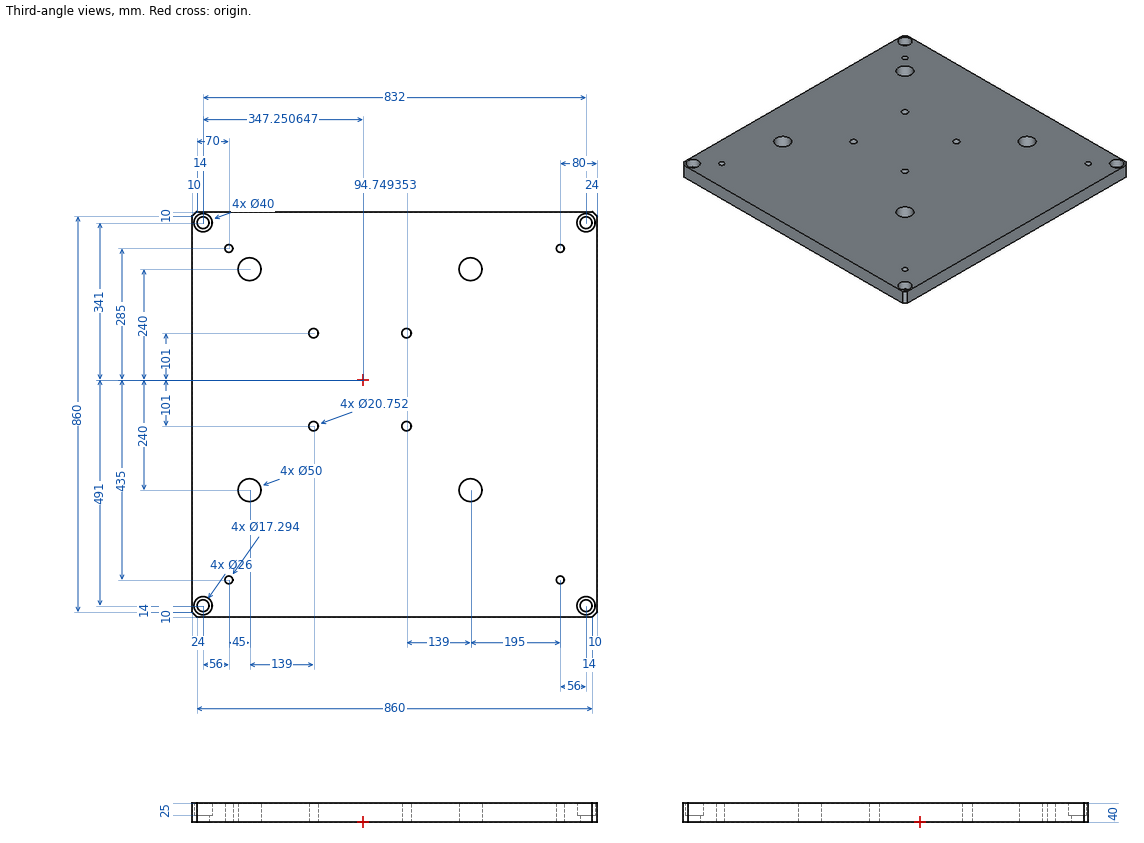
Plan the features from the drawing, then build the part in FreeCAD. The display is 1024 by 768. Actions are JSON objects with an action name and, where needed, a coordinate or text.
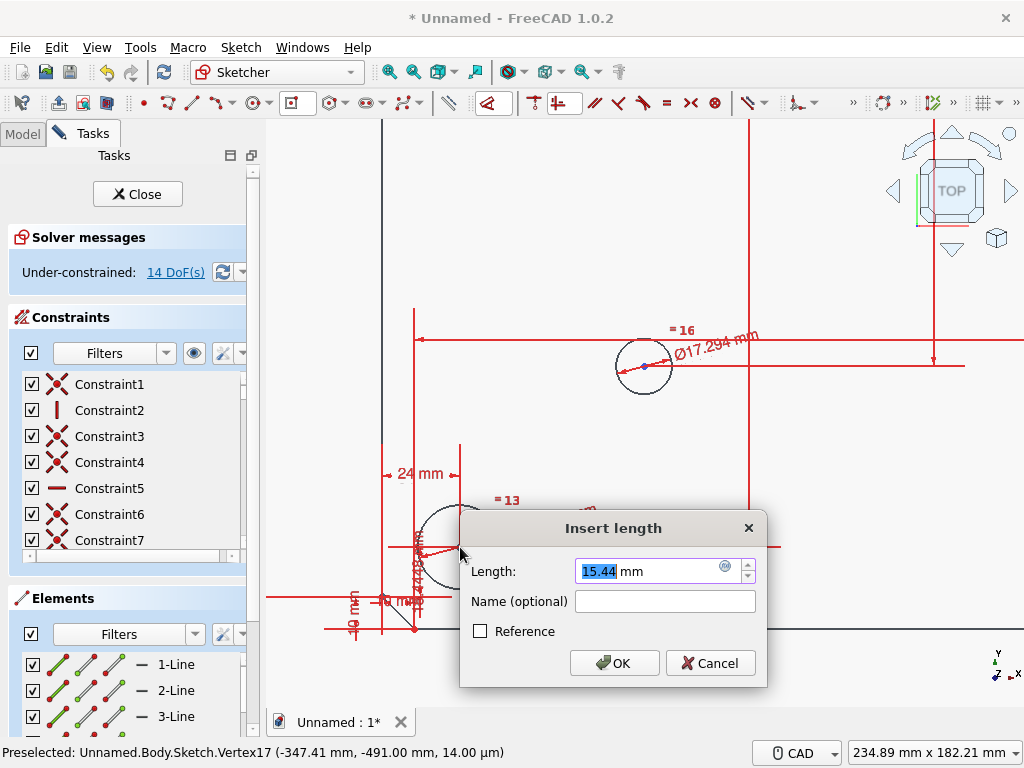
{"action": "type", "text": "14"}
{"action": "key", "text": "Return"}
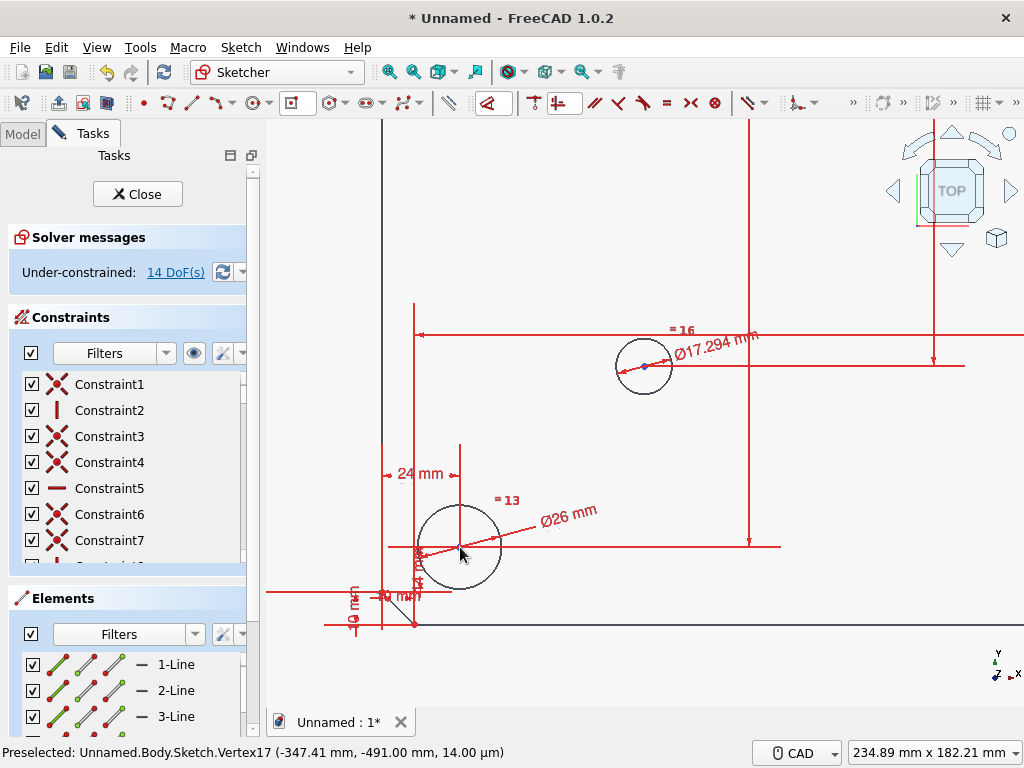
{"action": "scroll", "coordinate": [385, 602], "scroll_direction": "down", "scroll_amount": 10}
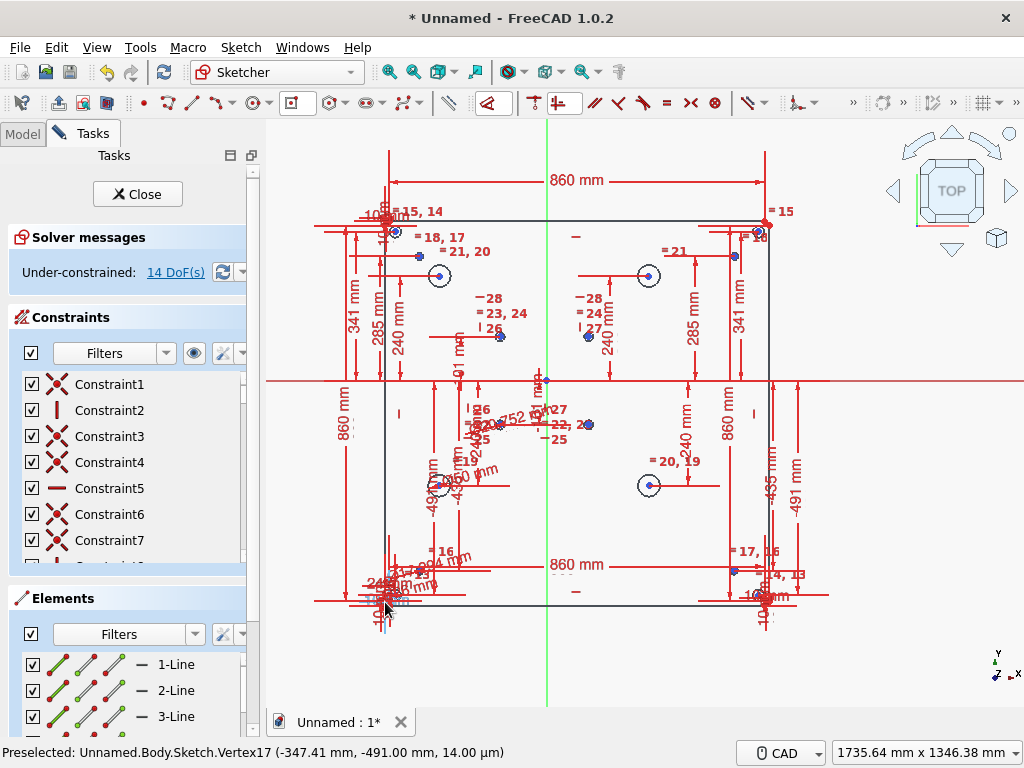
{"action": "scroll", "coordinate": [395, 595], "scroll_direction": "up", "scroll_amount": 3}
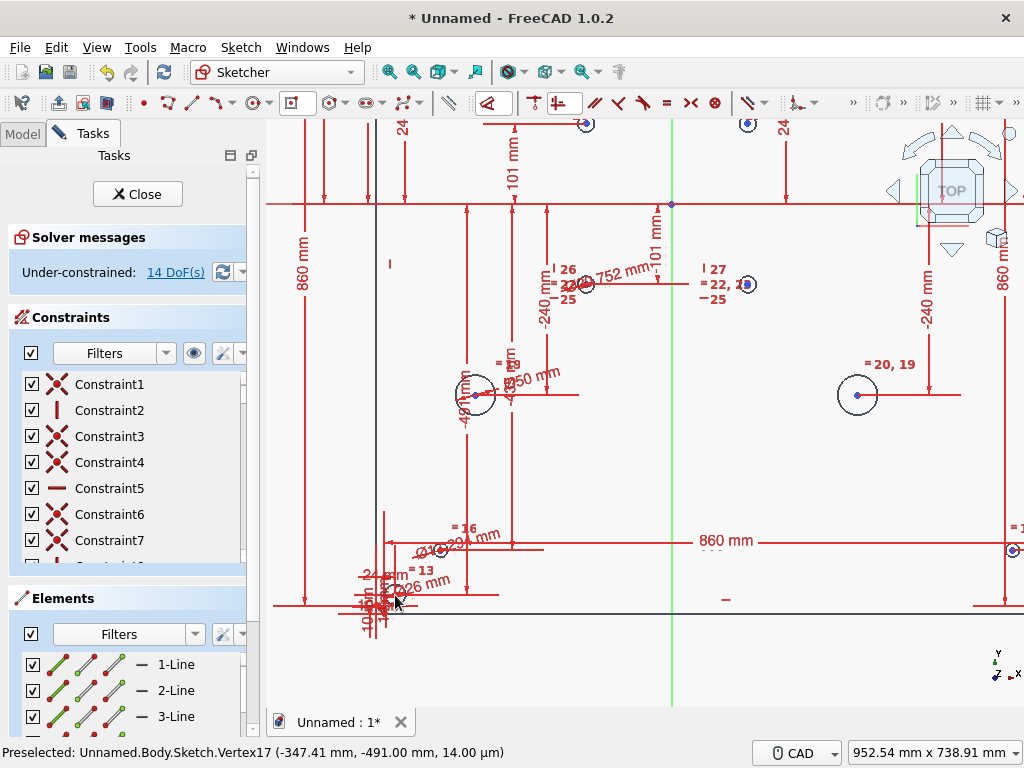
{"action": "left_click", "coordinate": [395, 595]}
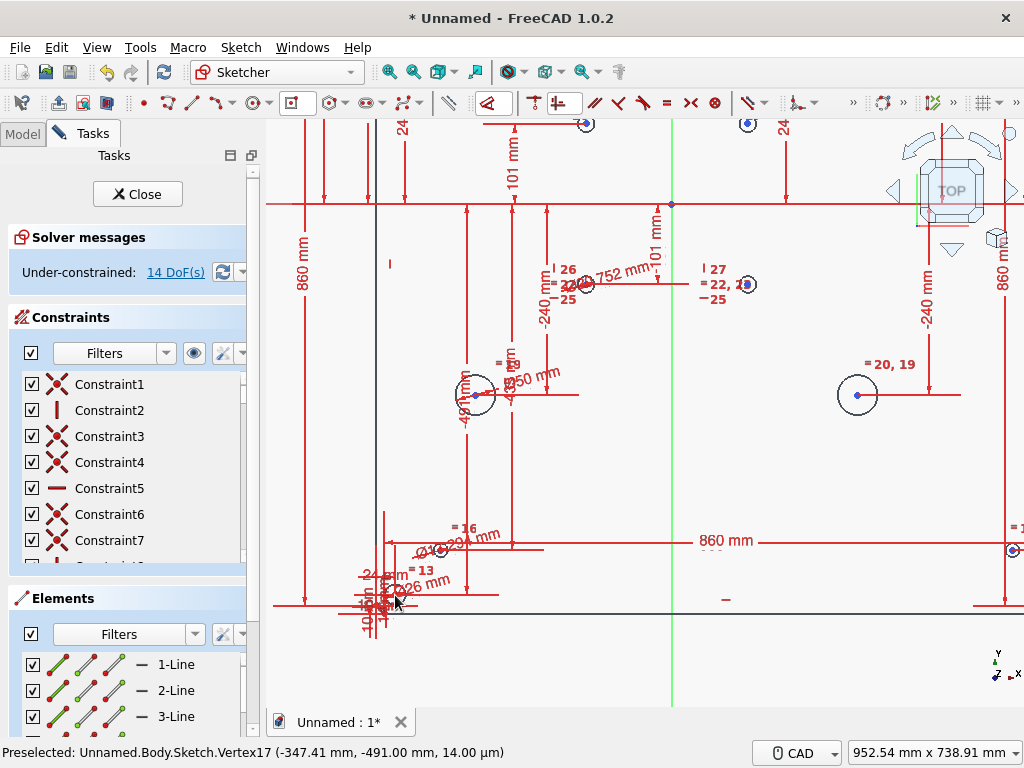
{"action": "left_click", "coordinate": [441, 550]}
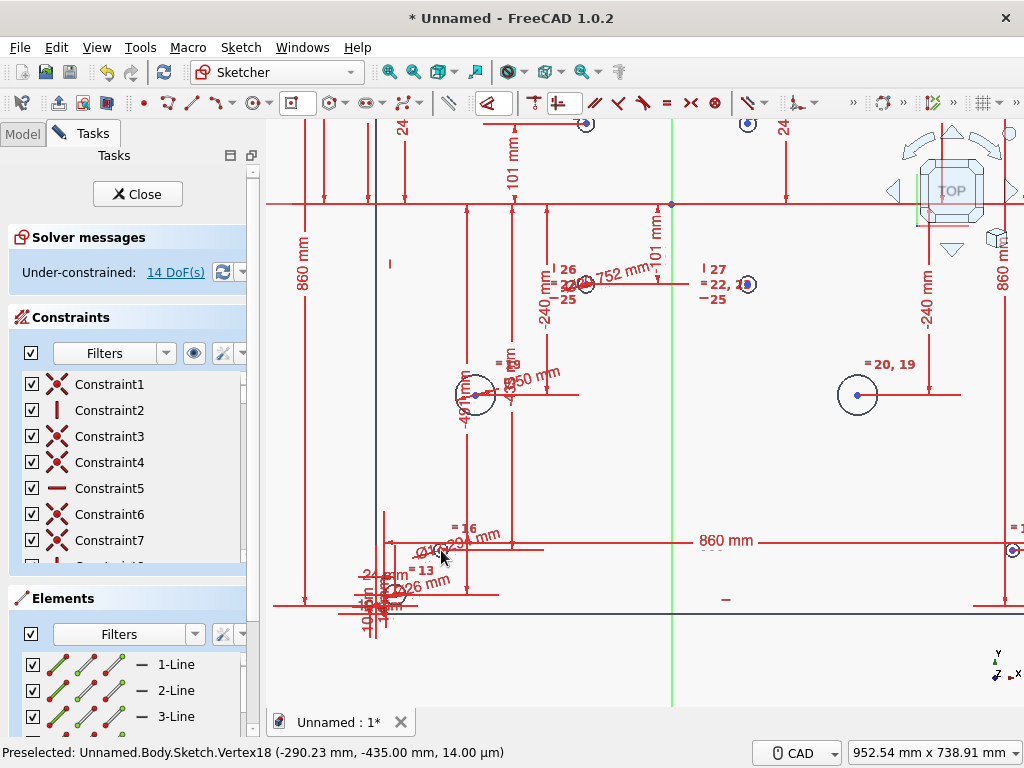
{"action": "left_click", "coordinate": [506, 104]}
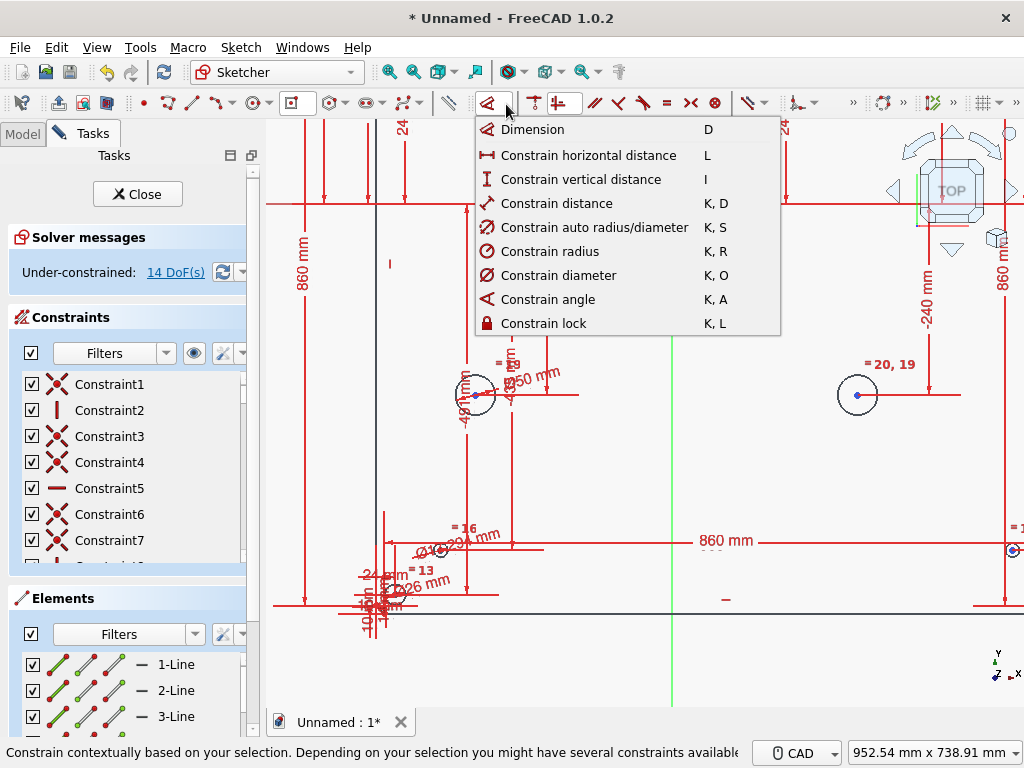
{"action": "left_click", "coordinate": [628, 155]}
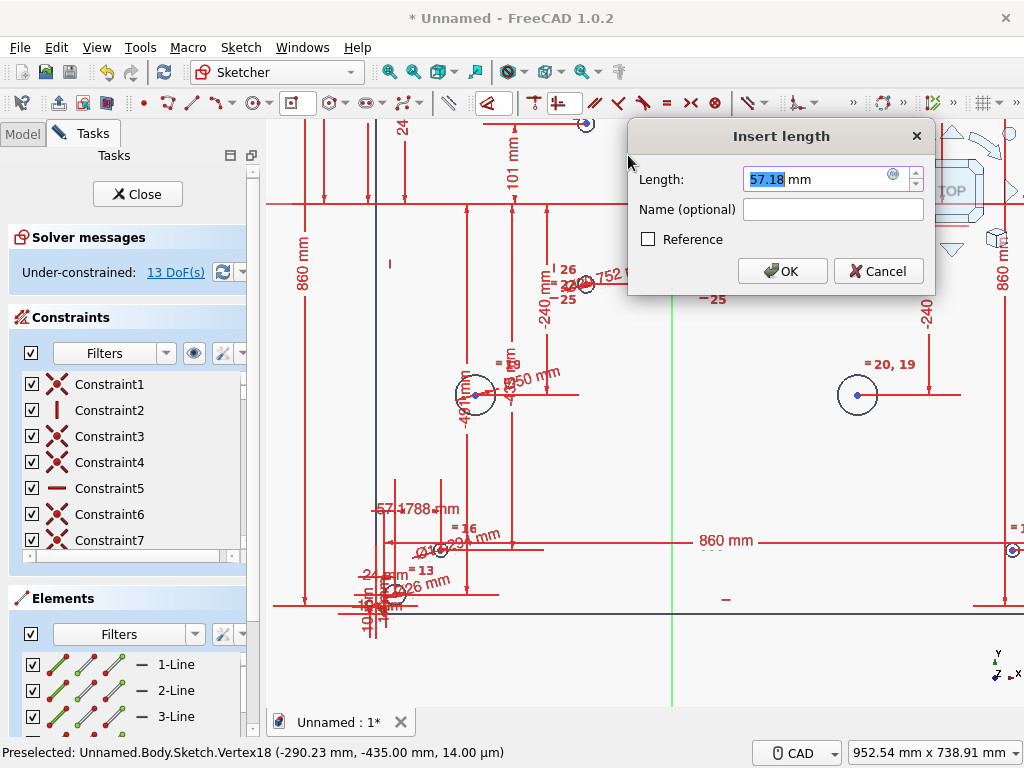
{"action": "type", "text": "56"}
{"action": "key", "text": "Return"}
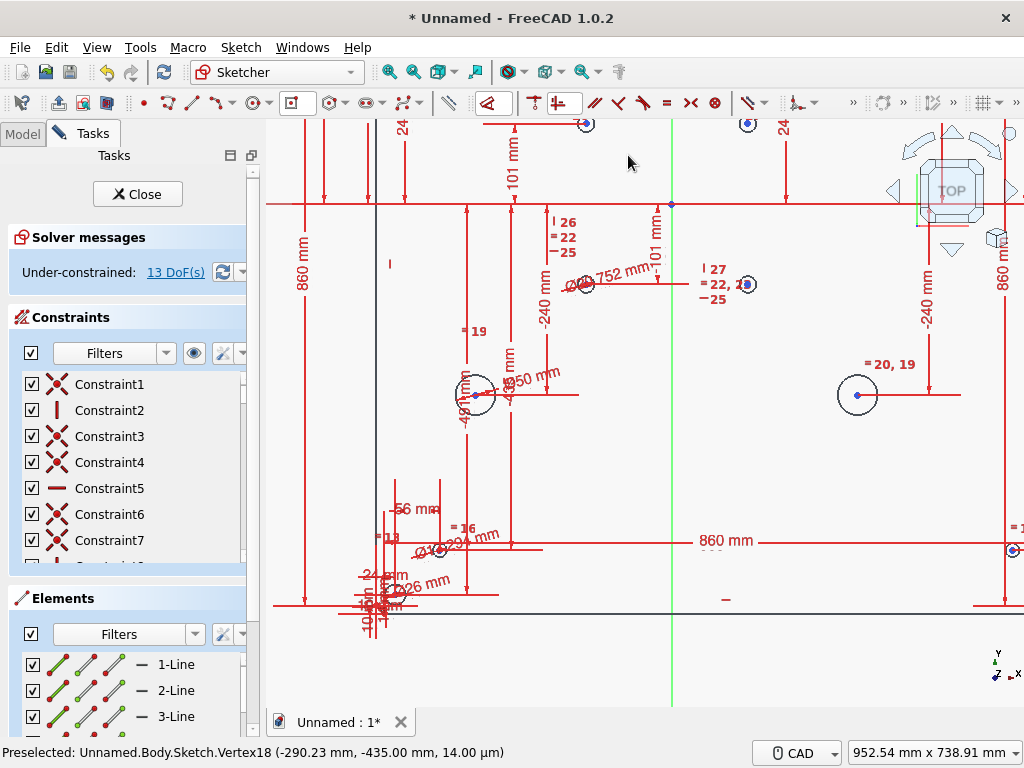
{"action": "left_click", "coordinate": [440, 550]}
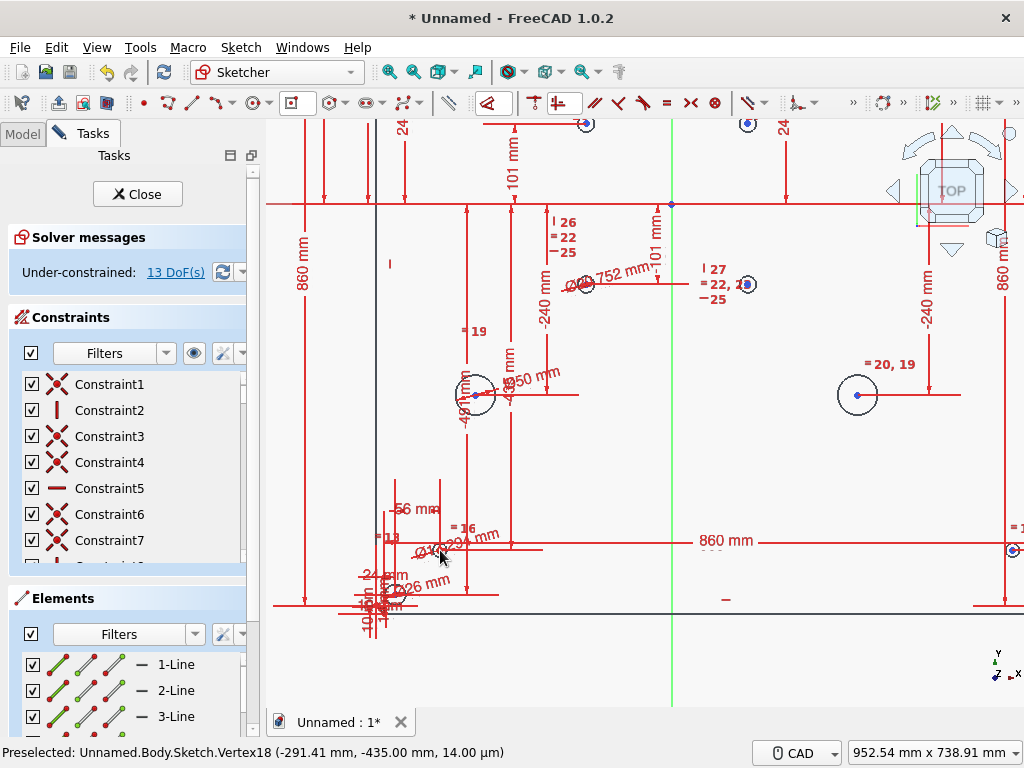
{"action": "left_click", "coordinate": [475, 395]}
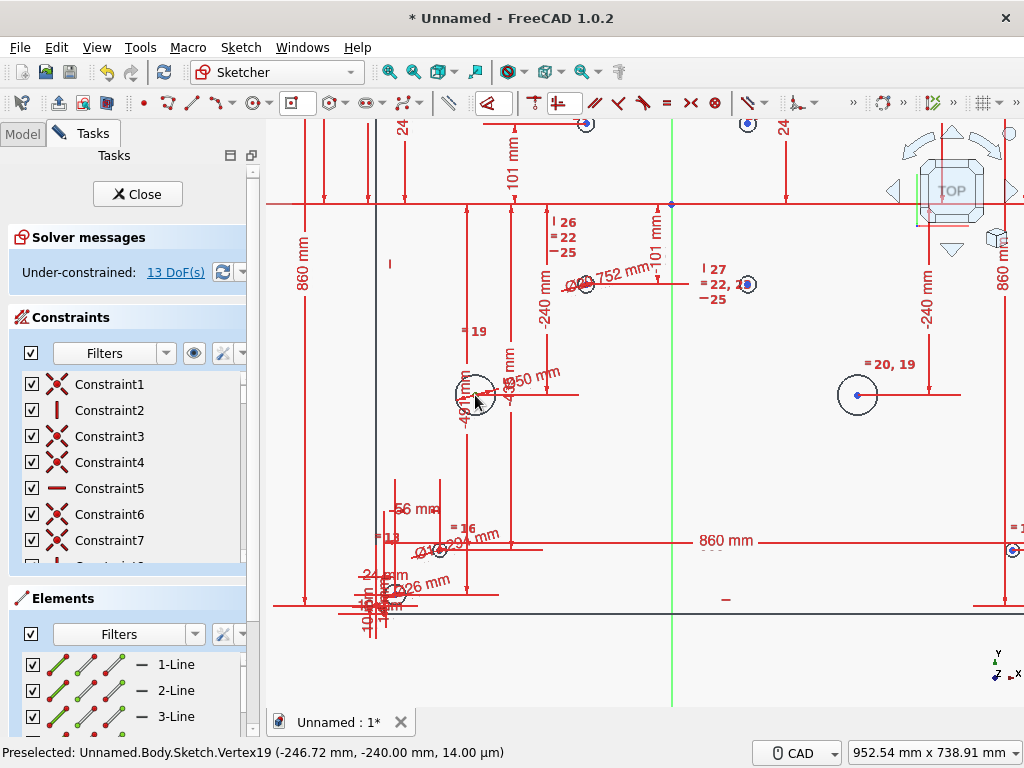
{"action": "key", "text": "l"}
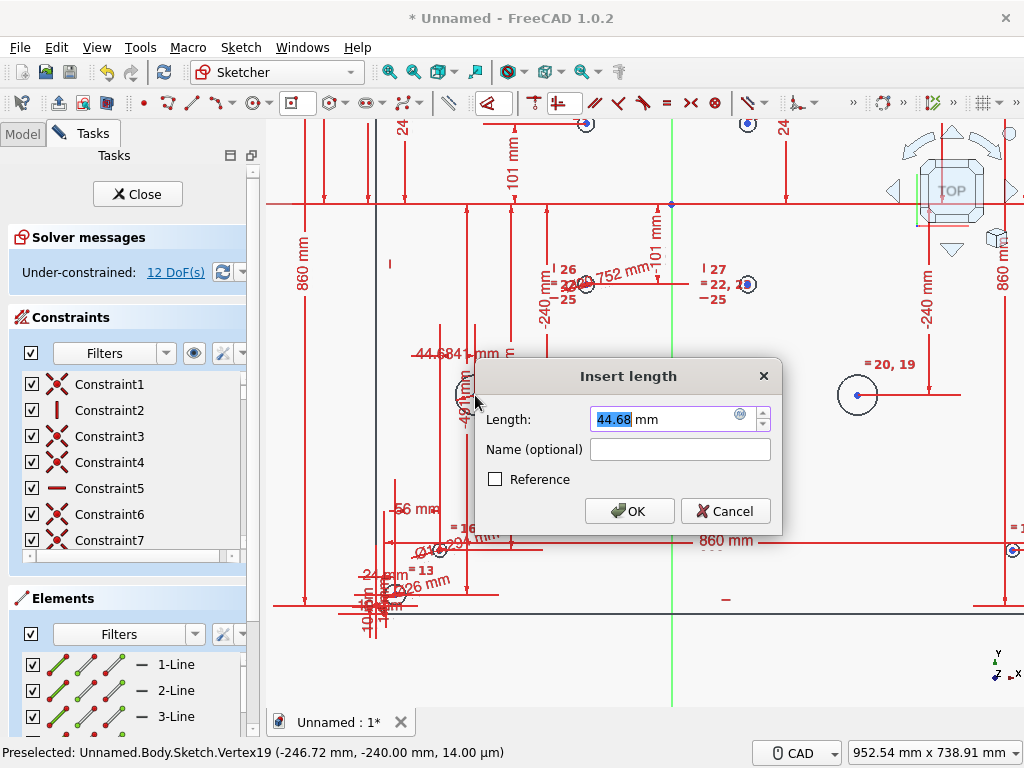
{"action": "type", "text": "45"}
{"action": "key", "text": "Return"}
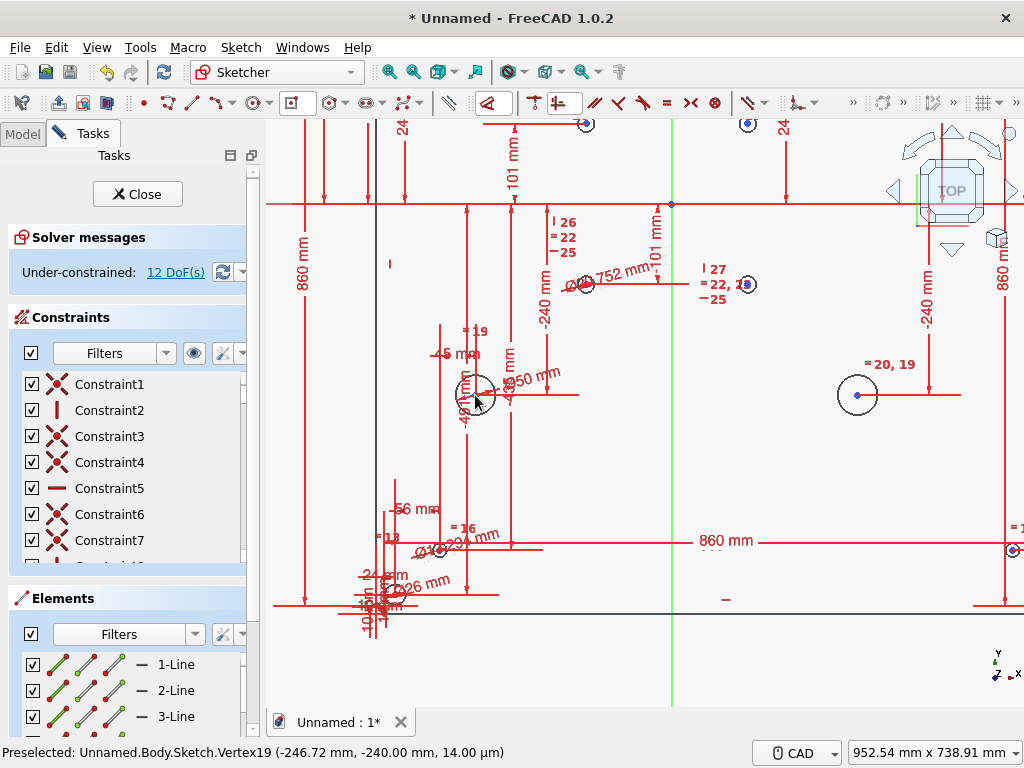
{"action": "scroll", "coordinate": [394, 594], "scroll_direction": "down", "scroll_amount": 3}